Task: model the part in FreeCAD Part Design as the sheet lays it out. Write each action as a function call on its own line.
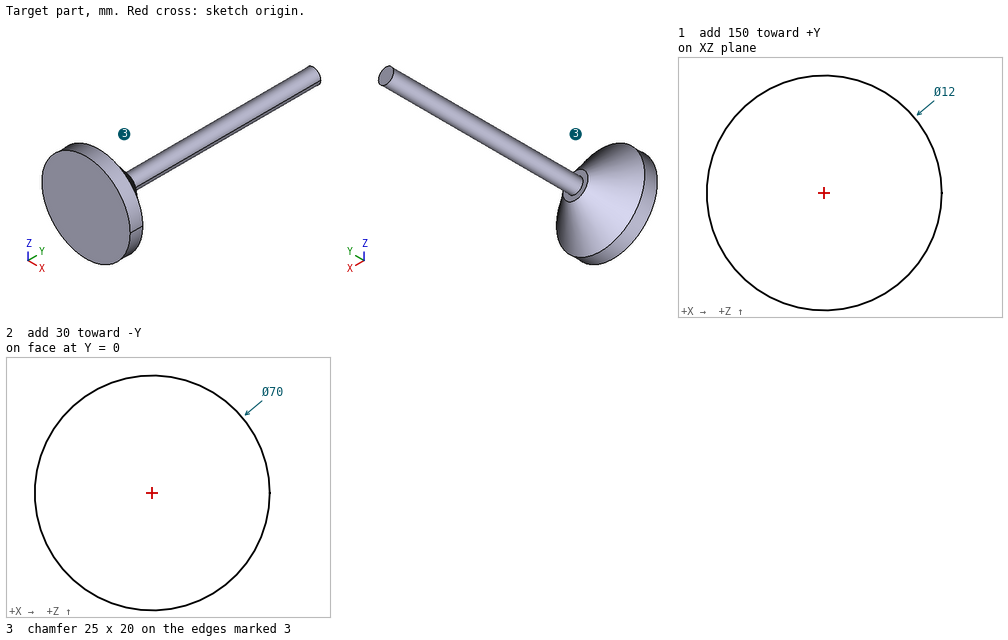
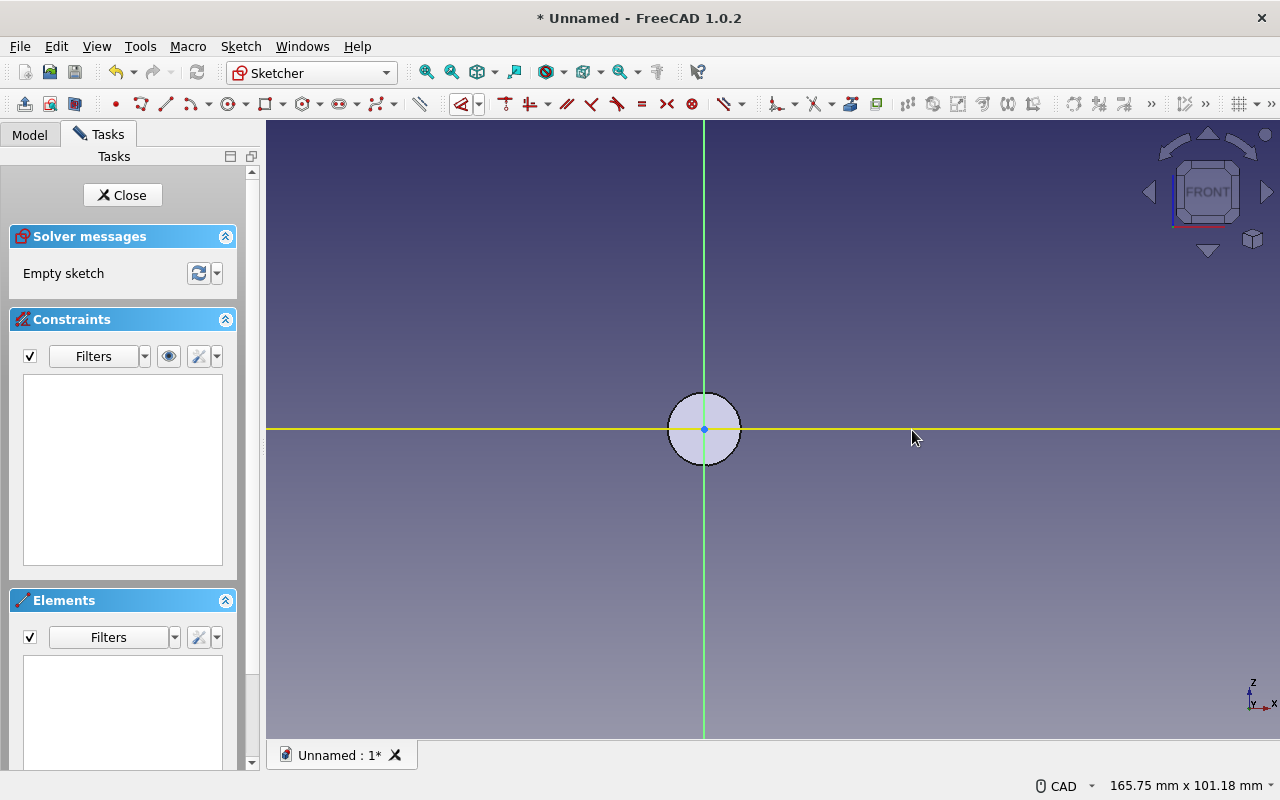
click(228, 104)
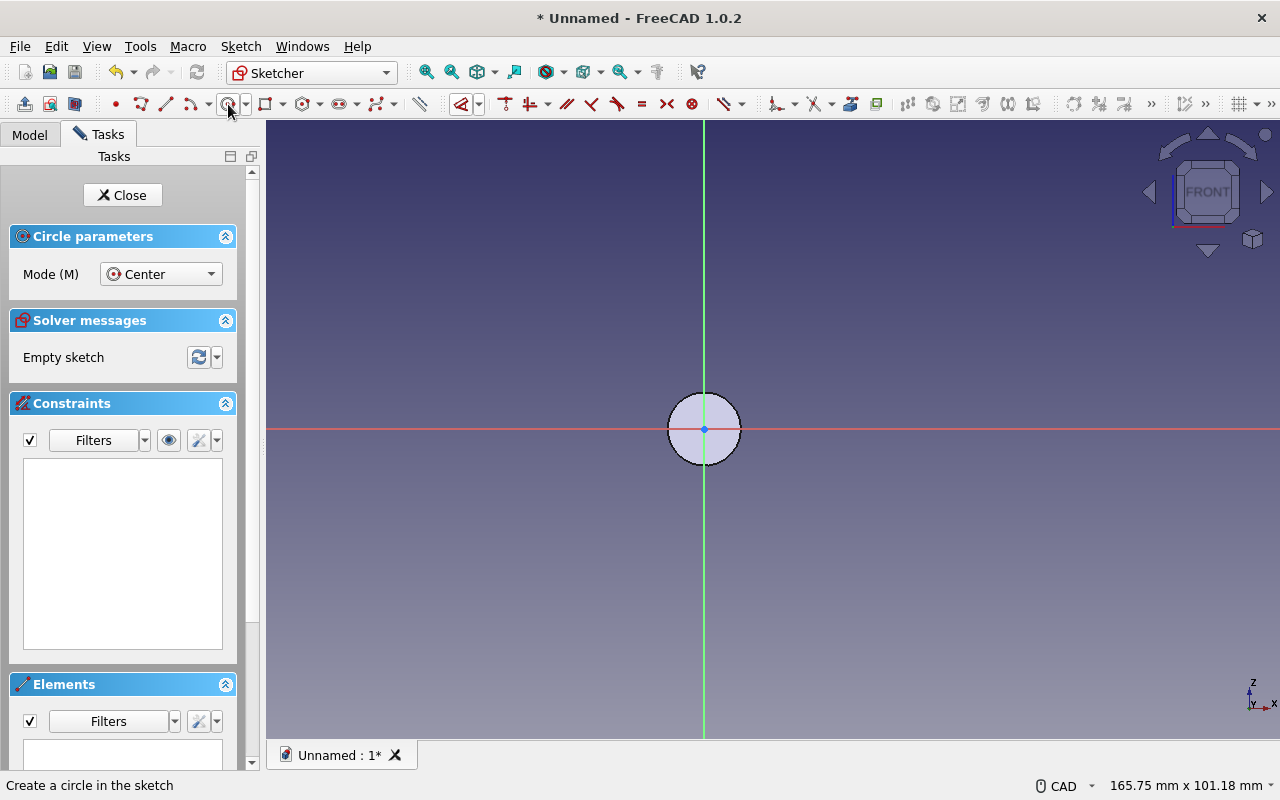
click(704, 429)
click(856, 278)
key(Escape)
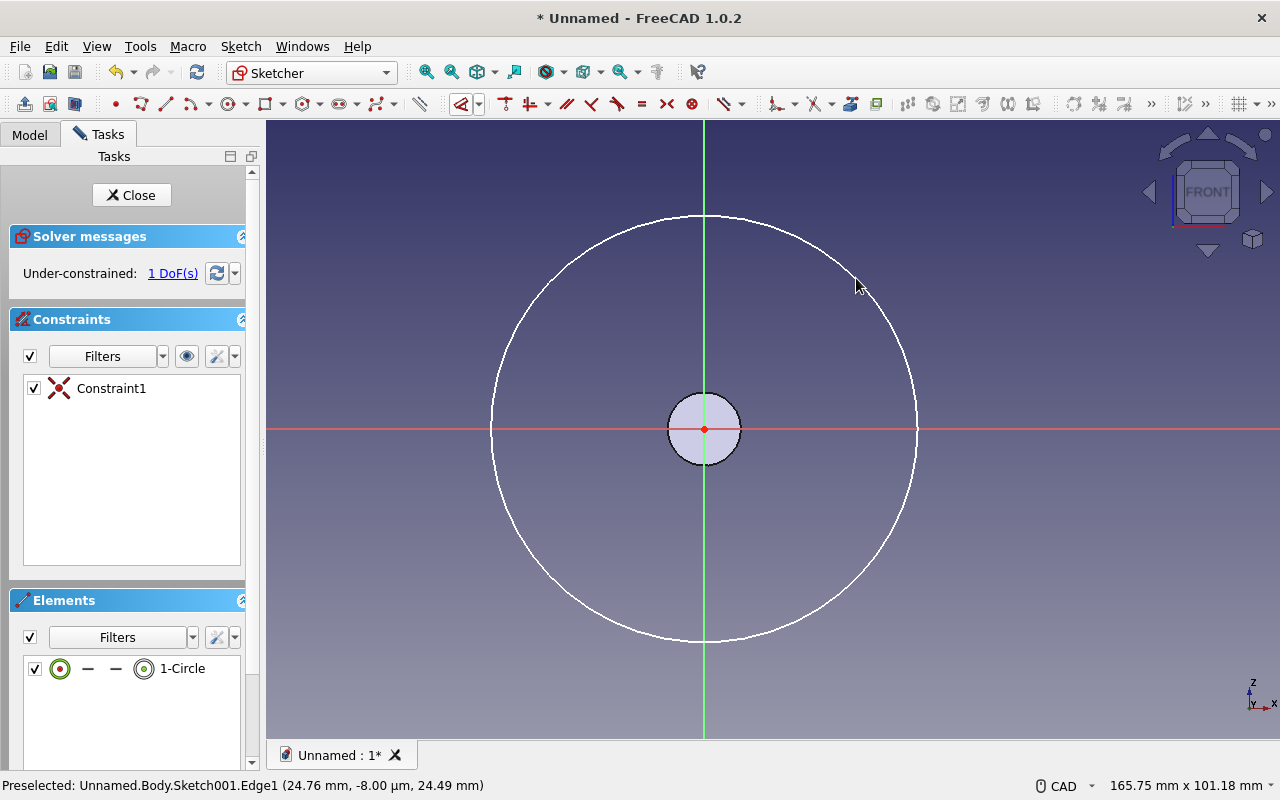
click(855, 278)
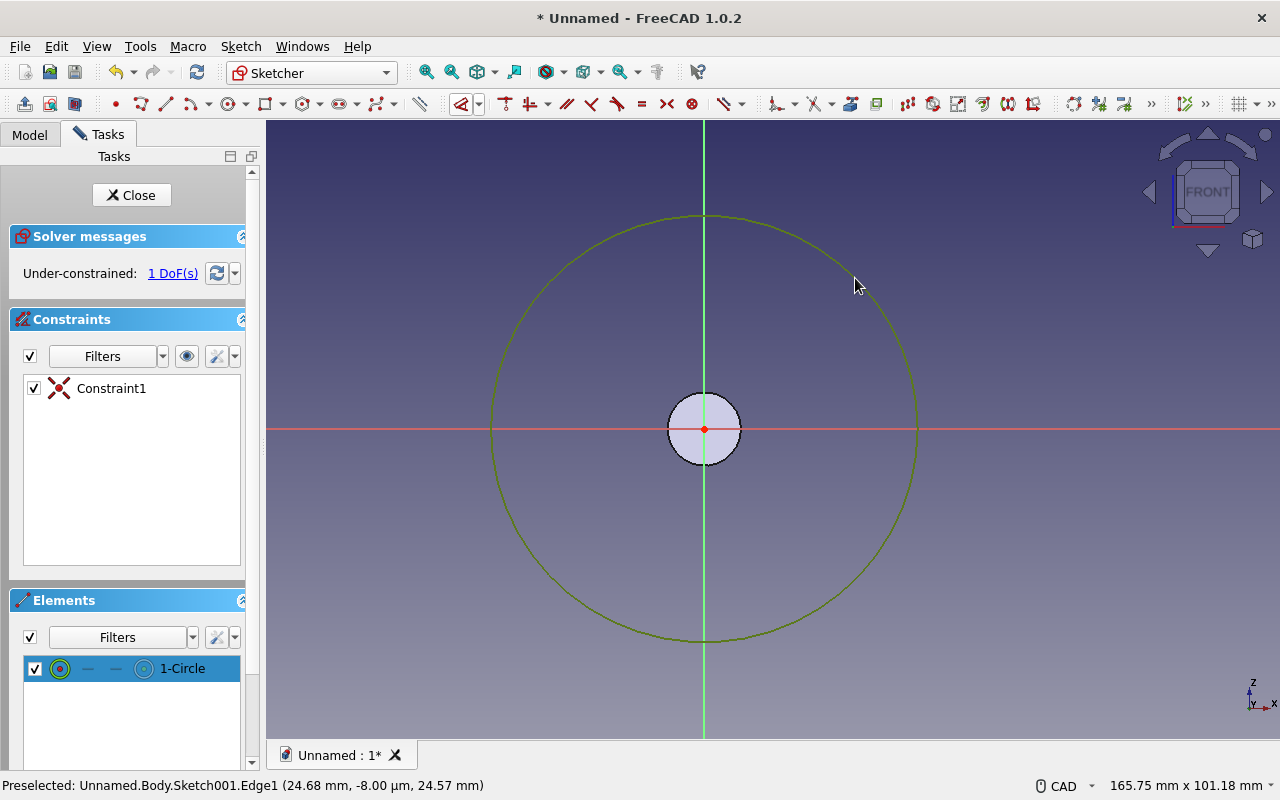
key(k)
key(o)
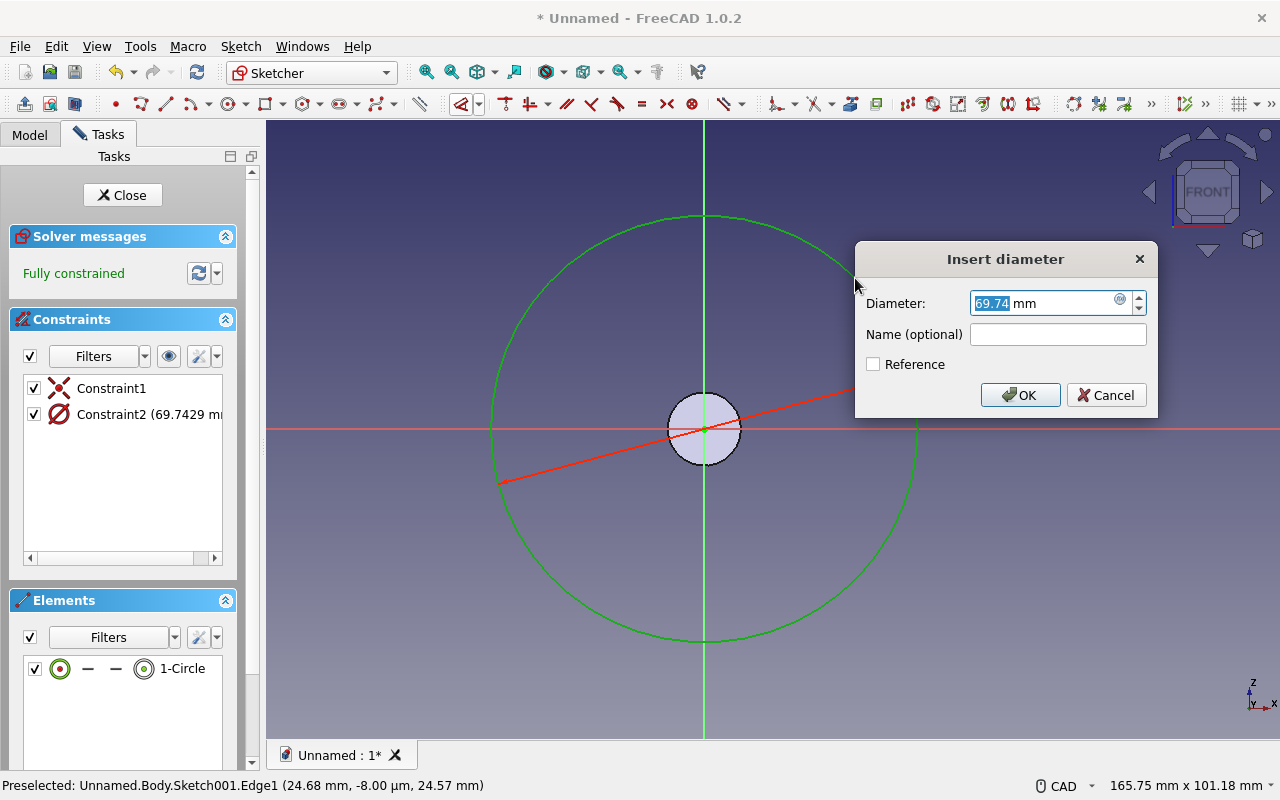
text(70)
key(Return)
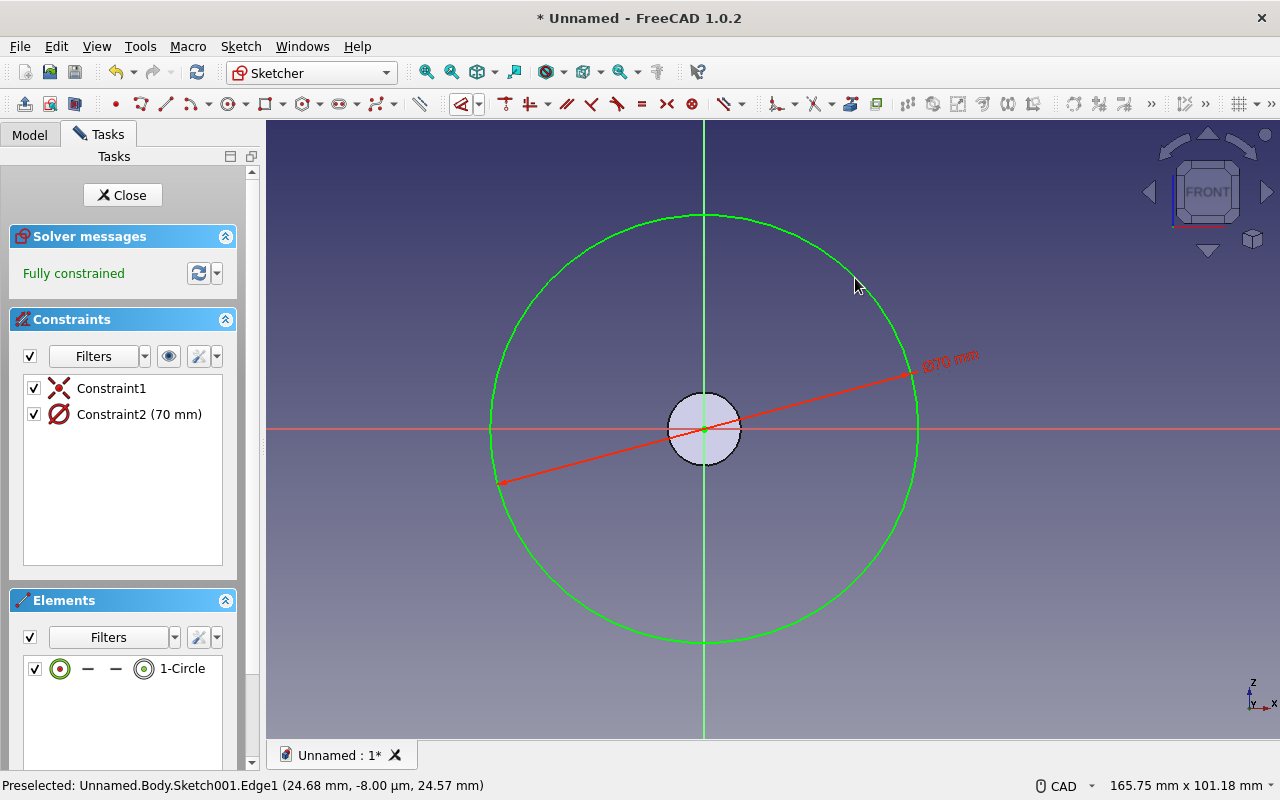
click(123, 195)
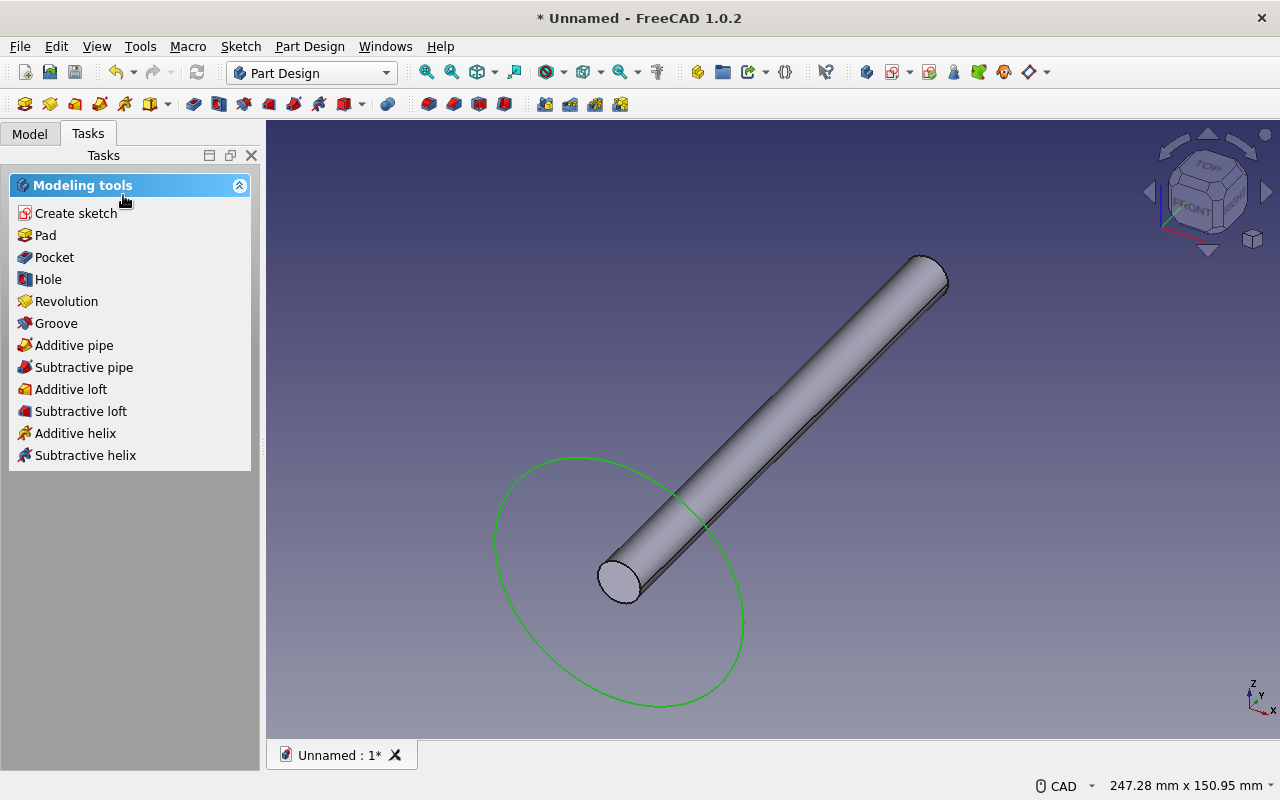
click(25, 104)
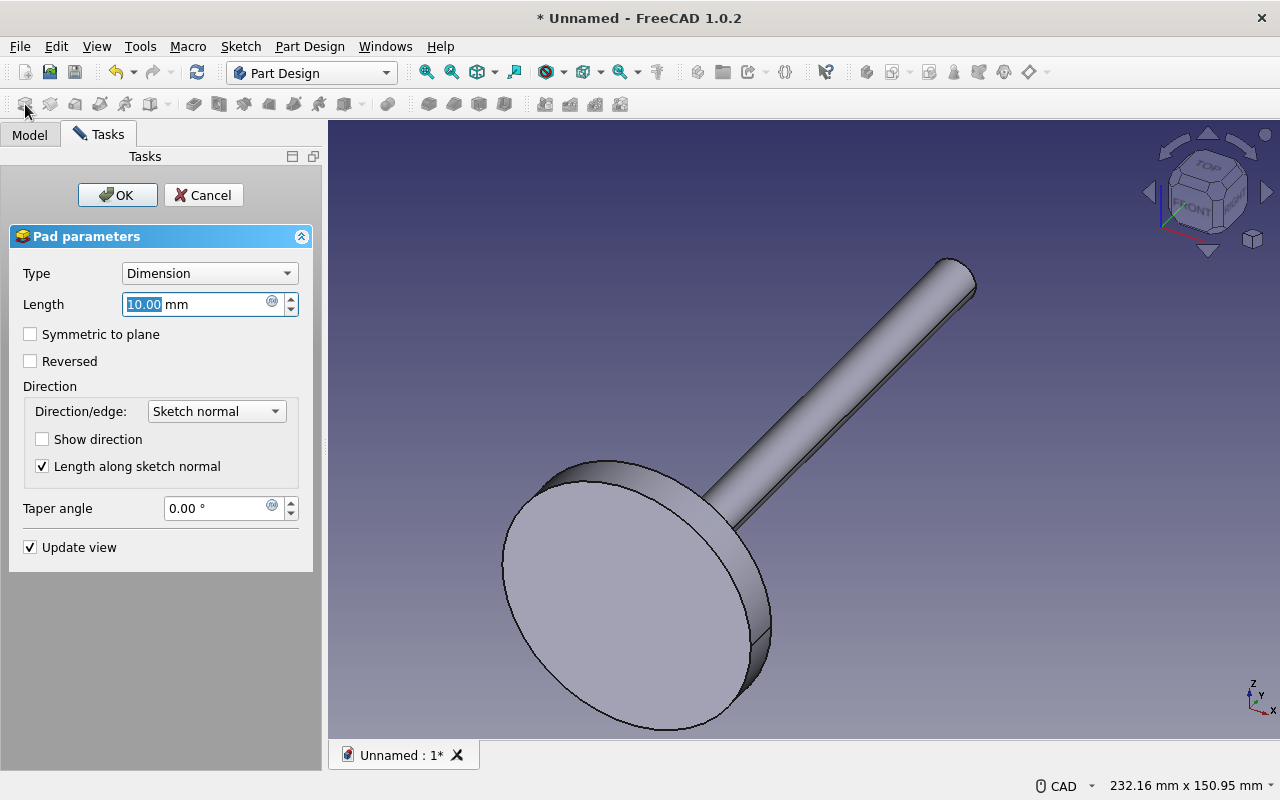
text(30)
key(Tab)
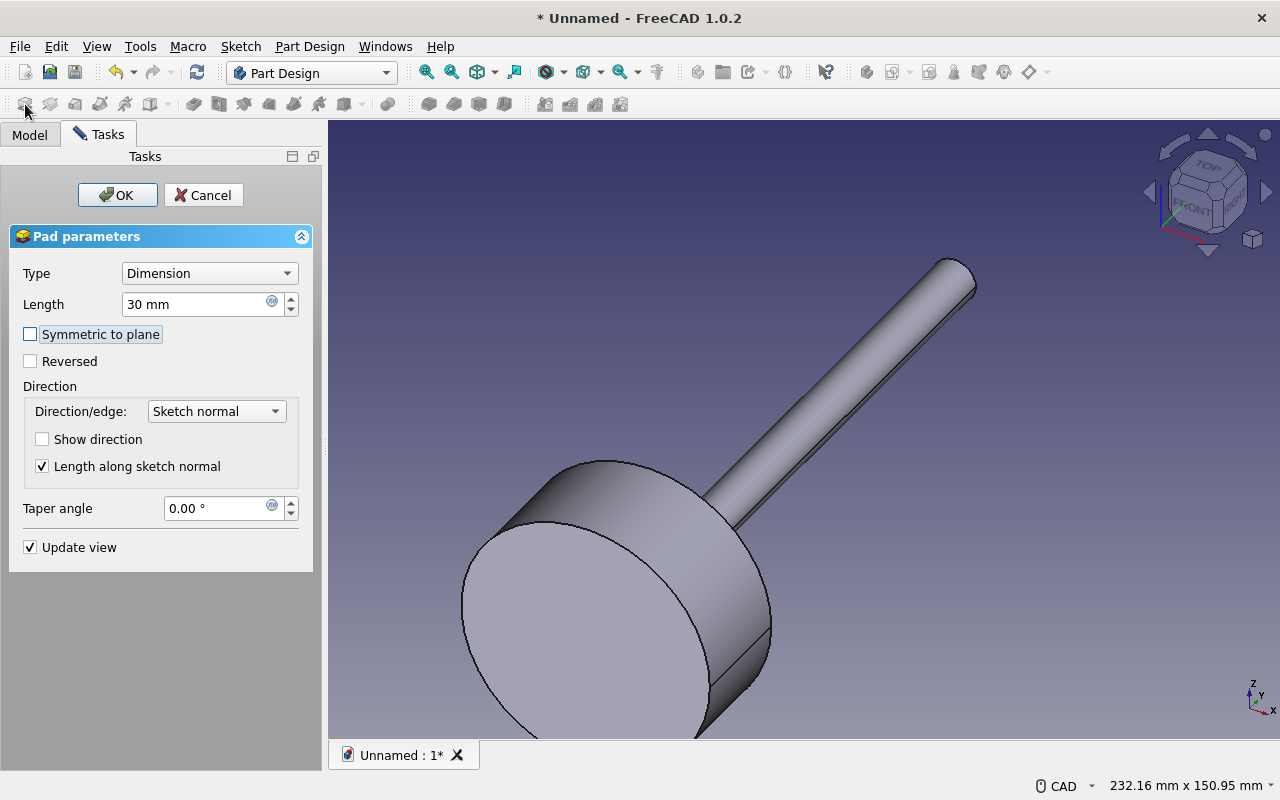
click(118, 195)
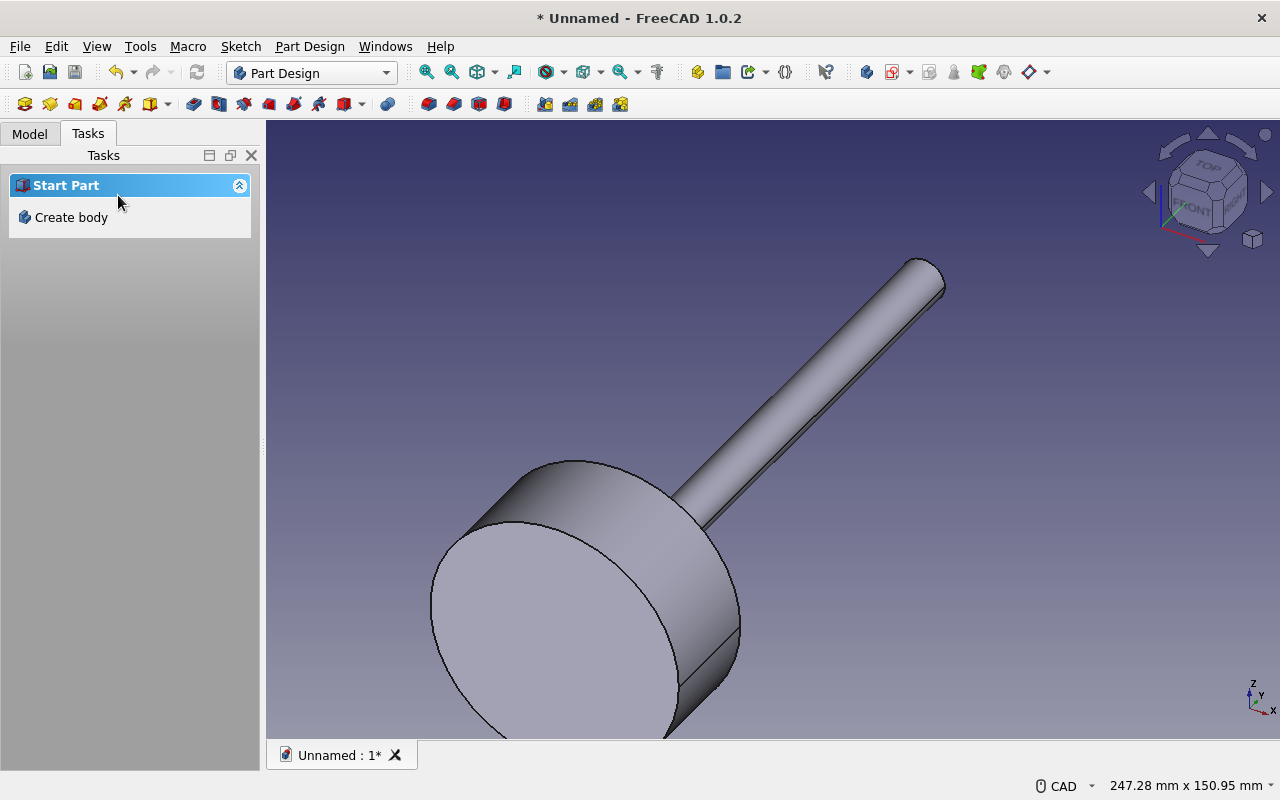
click(427, 72)